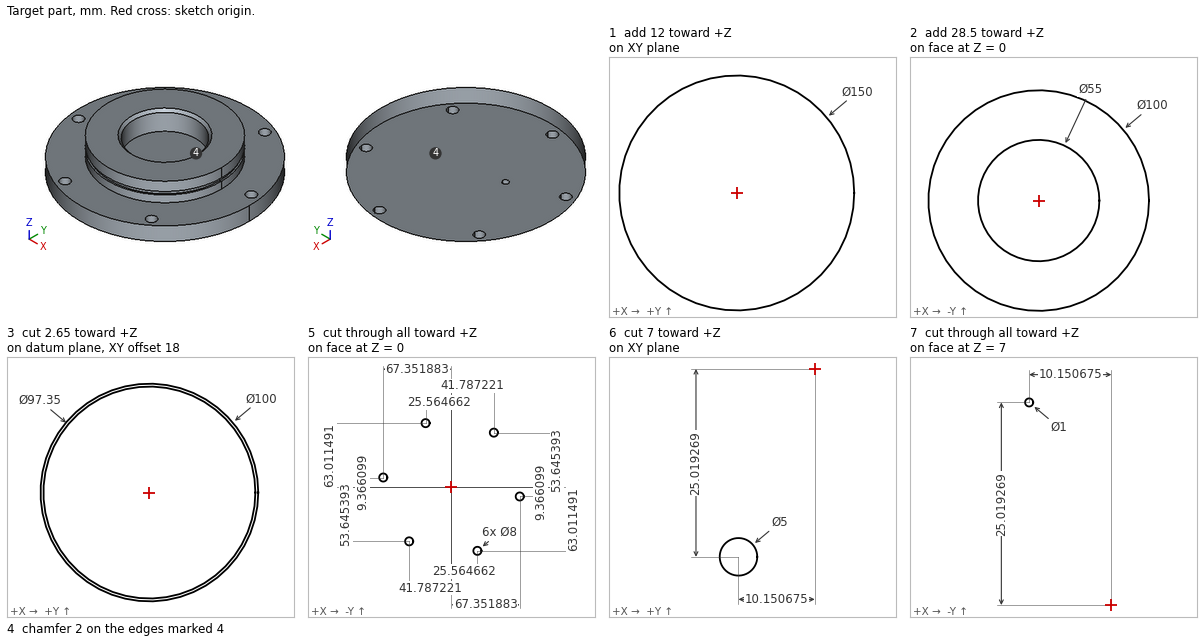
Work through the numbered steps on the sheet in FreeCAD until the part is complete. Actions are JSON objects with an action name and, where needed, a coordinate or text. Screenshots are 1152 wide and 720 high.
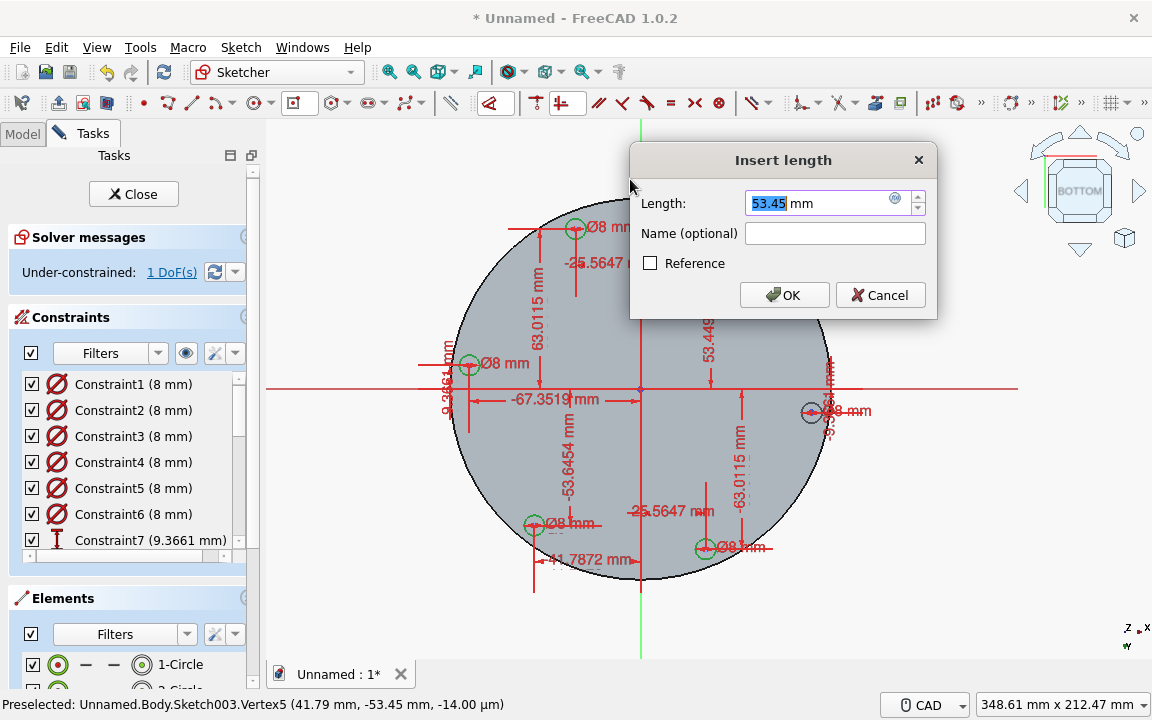
{"action": "type", "text": "53.645393"}
{"action": "key", "text": "Return"}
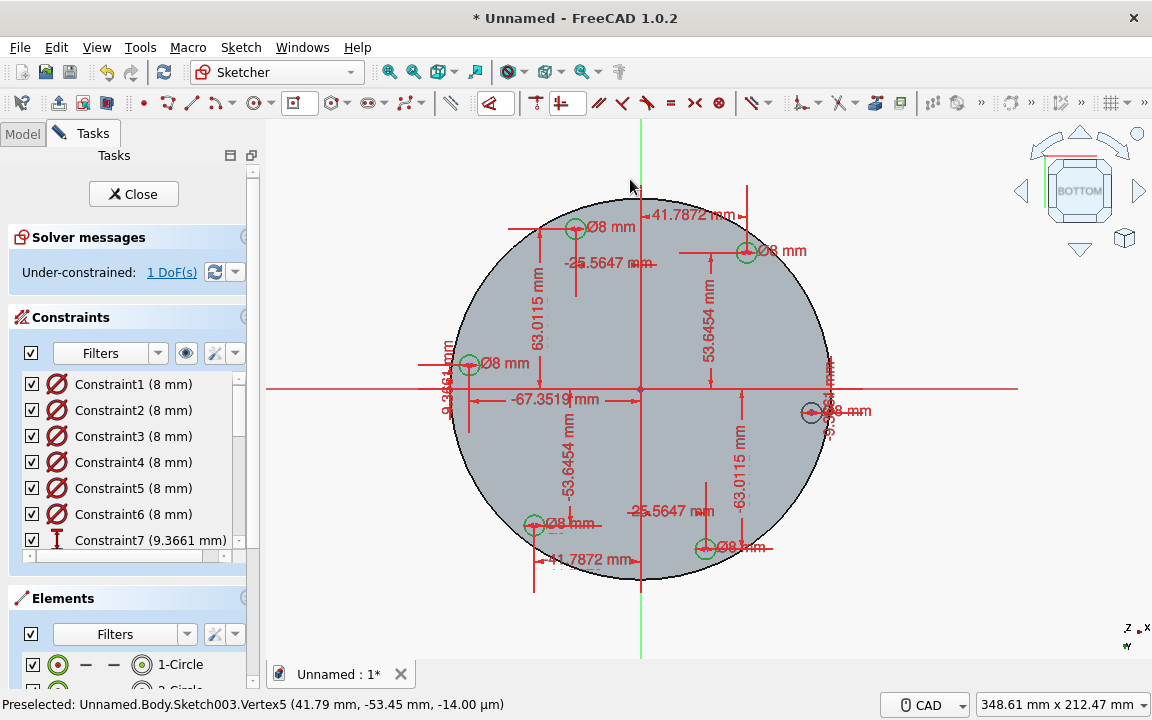
{"action": "left_click", "coordinate": [812, 413]}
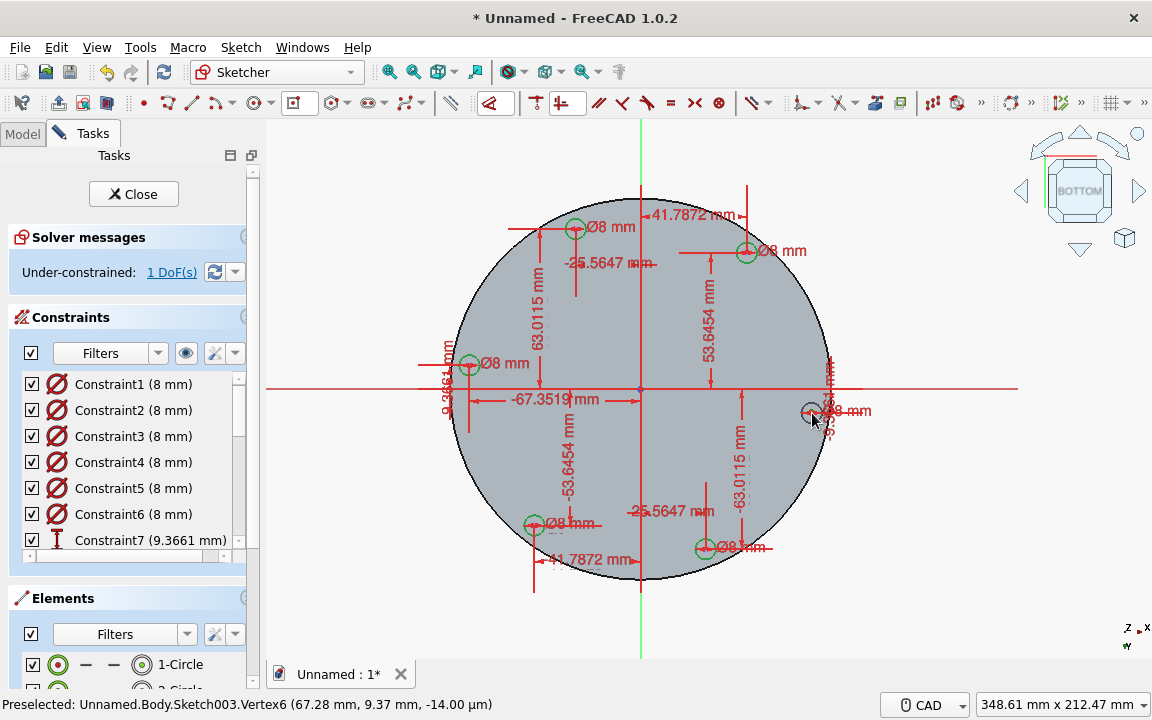
{"action": "key", "text": "l"}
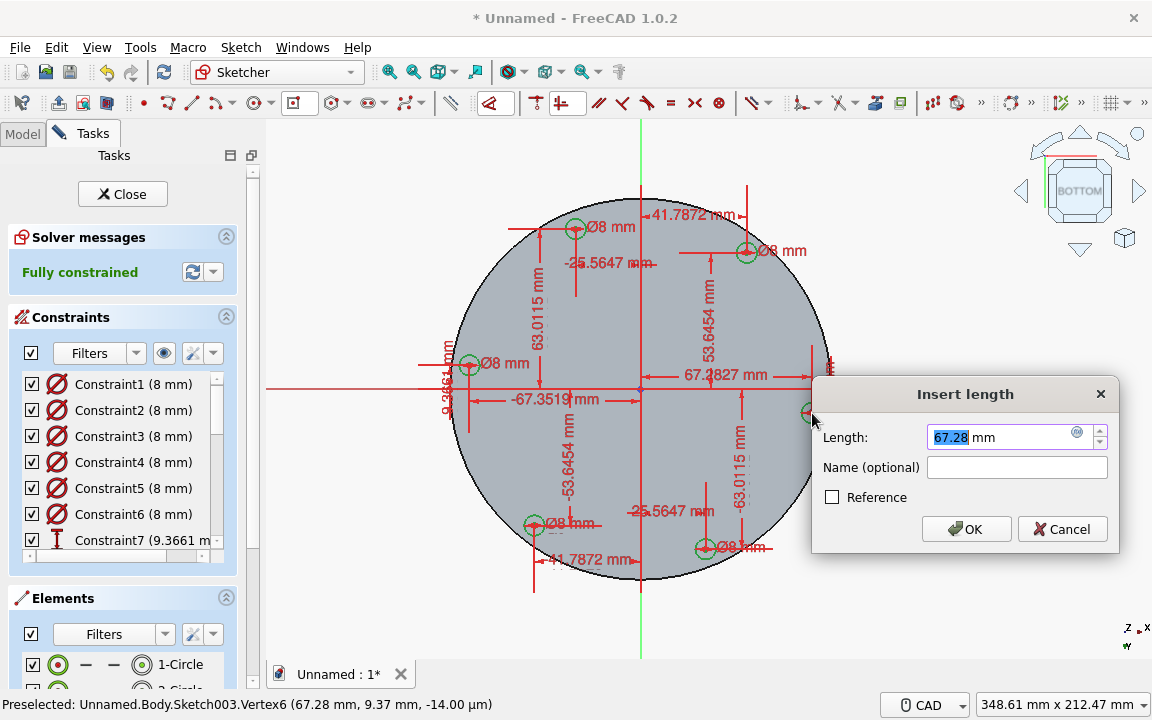
{"action": "type", "text": "67.351883"}
{"action": "key", "text": "Return"}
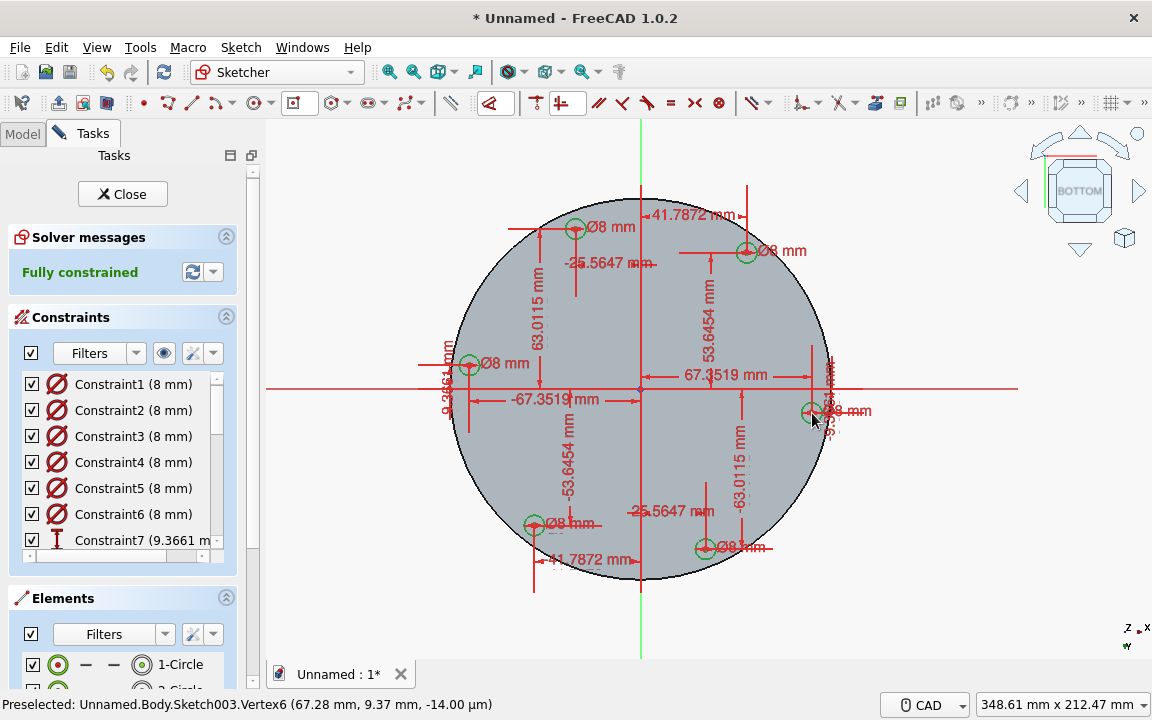
{"action": "left_click", "coordinate": [123, 194]}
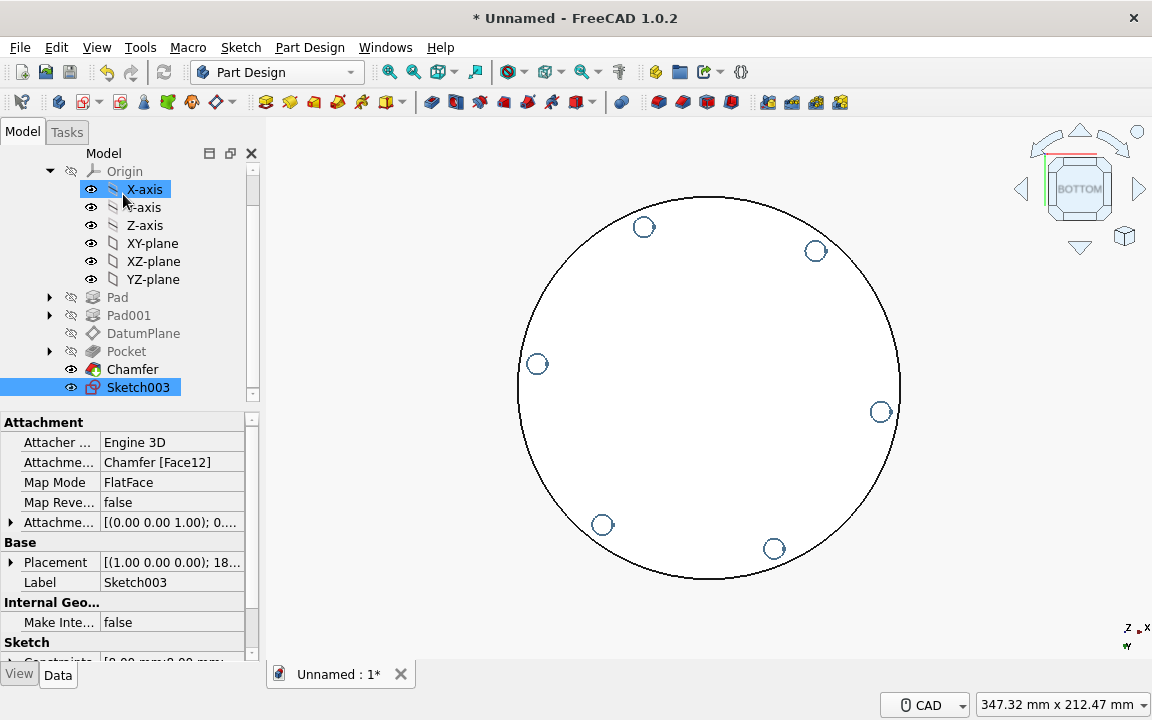
{"action": "left_click", "coordinate": [432, 102]}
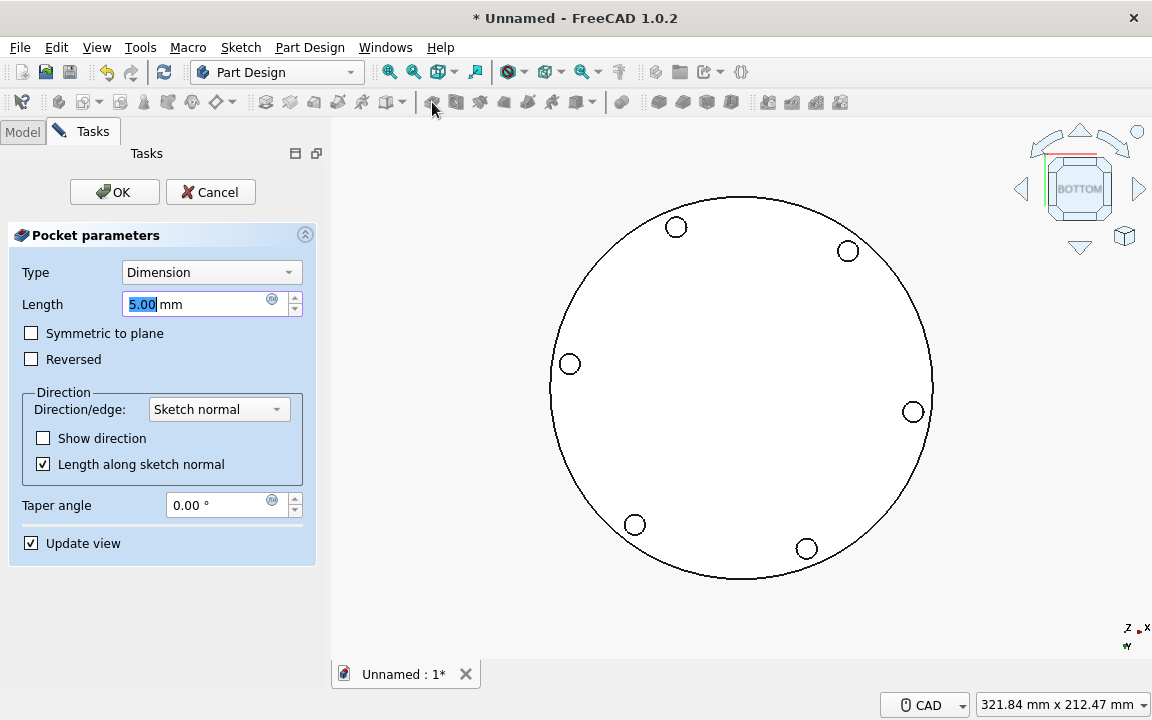
{"action": "left_click", "coordinate": [212, 272]}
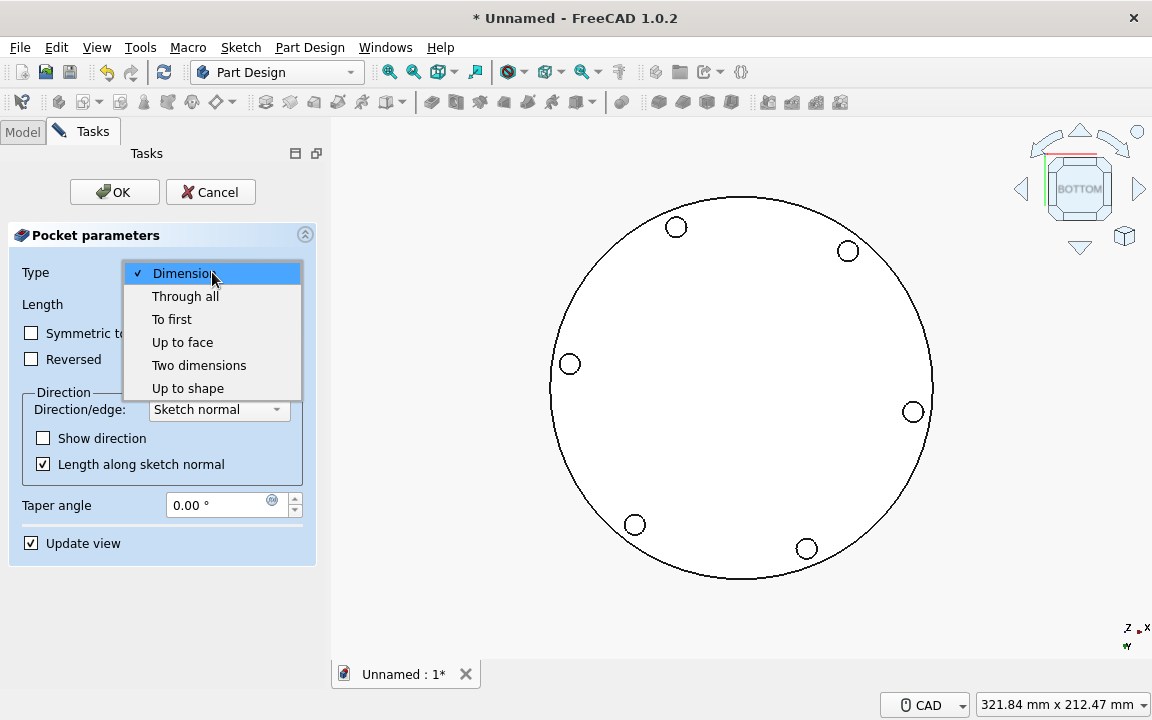
{"action": "left_click", "coordinate": [212, 296]}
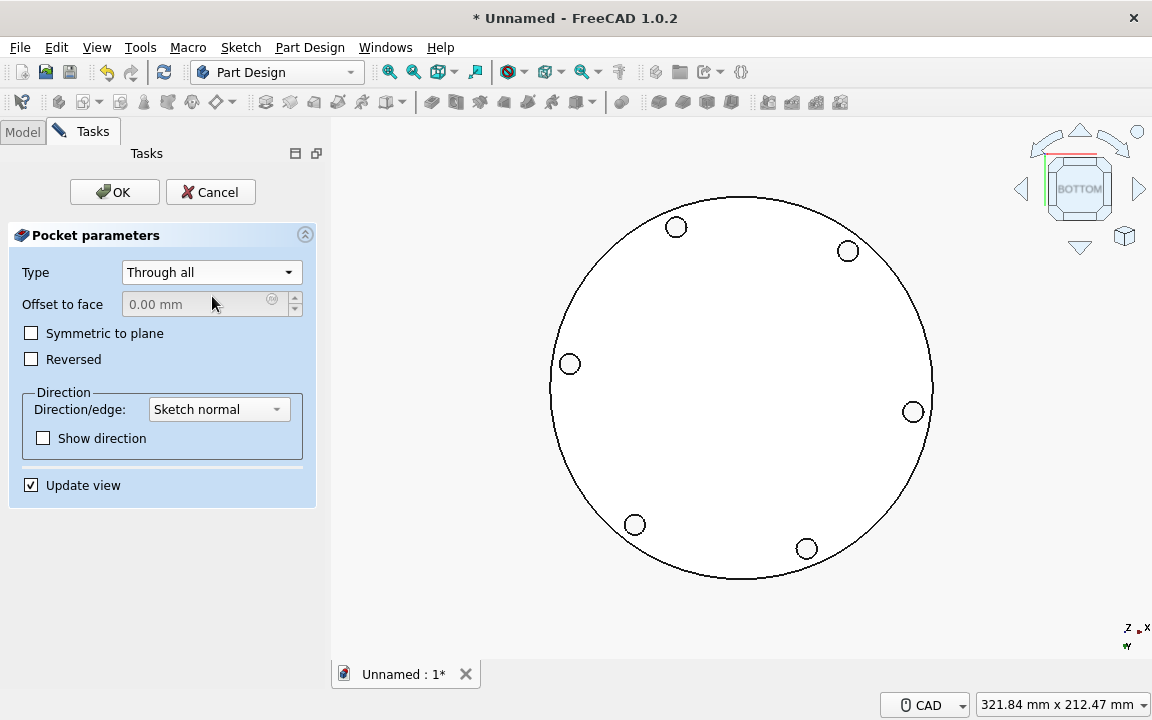
{"action": "left_click", "coordinate": [115, 192]}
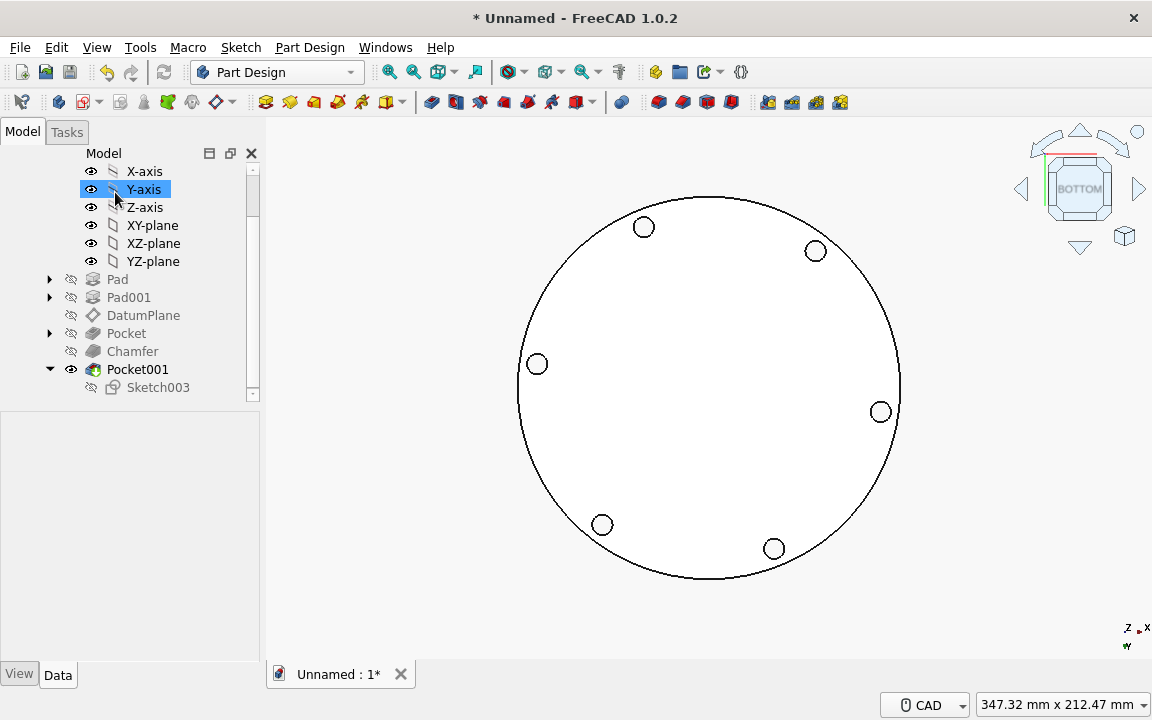
{"action": "left_click", "coordinate": [84, 102]}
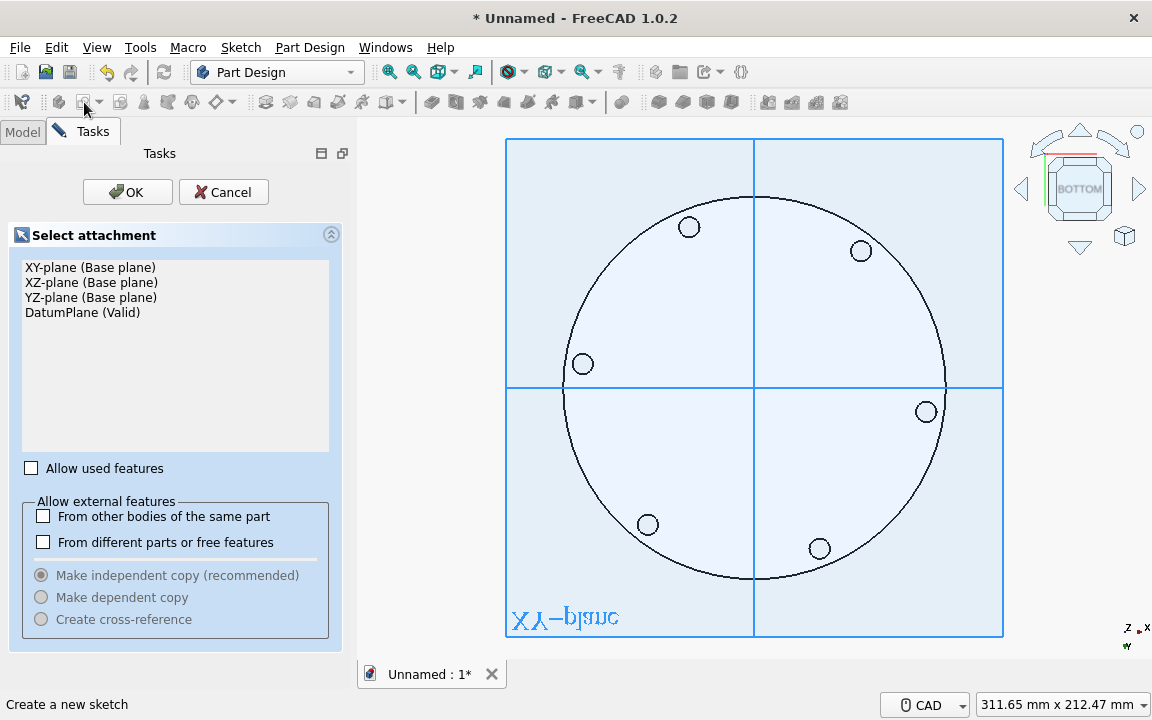
{"action": "left_click", "coordinate": [82, 268]}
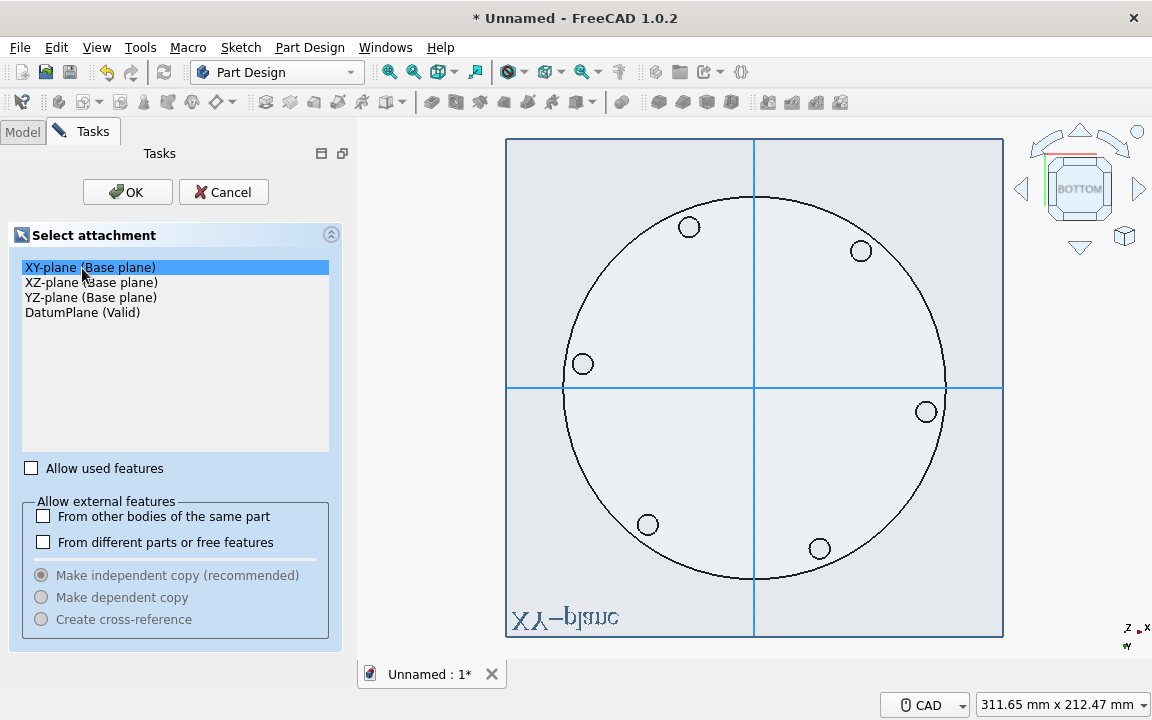
{"action": "left_click", "coordinate": [128, 192]}